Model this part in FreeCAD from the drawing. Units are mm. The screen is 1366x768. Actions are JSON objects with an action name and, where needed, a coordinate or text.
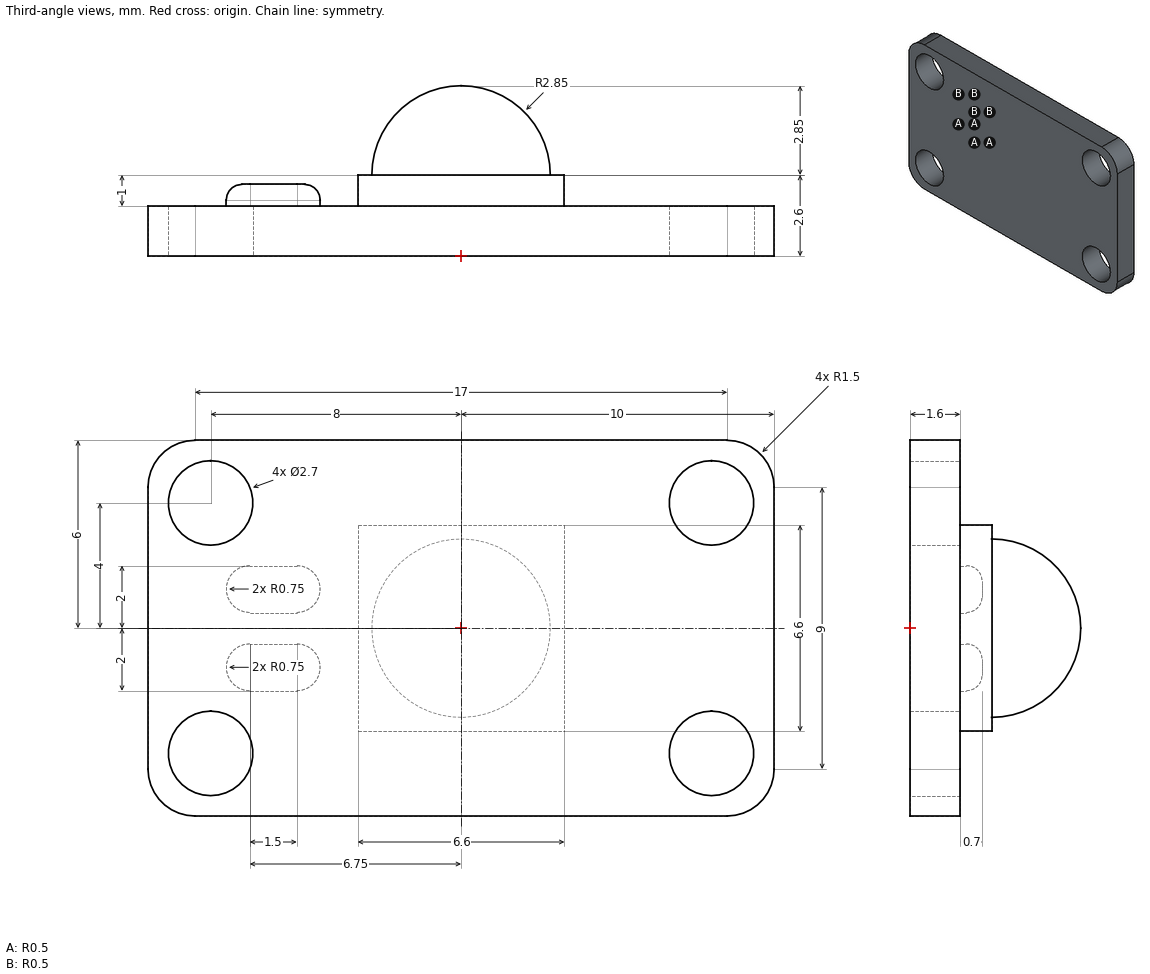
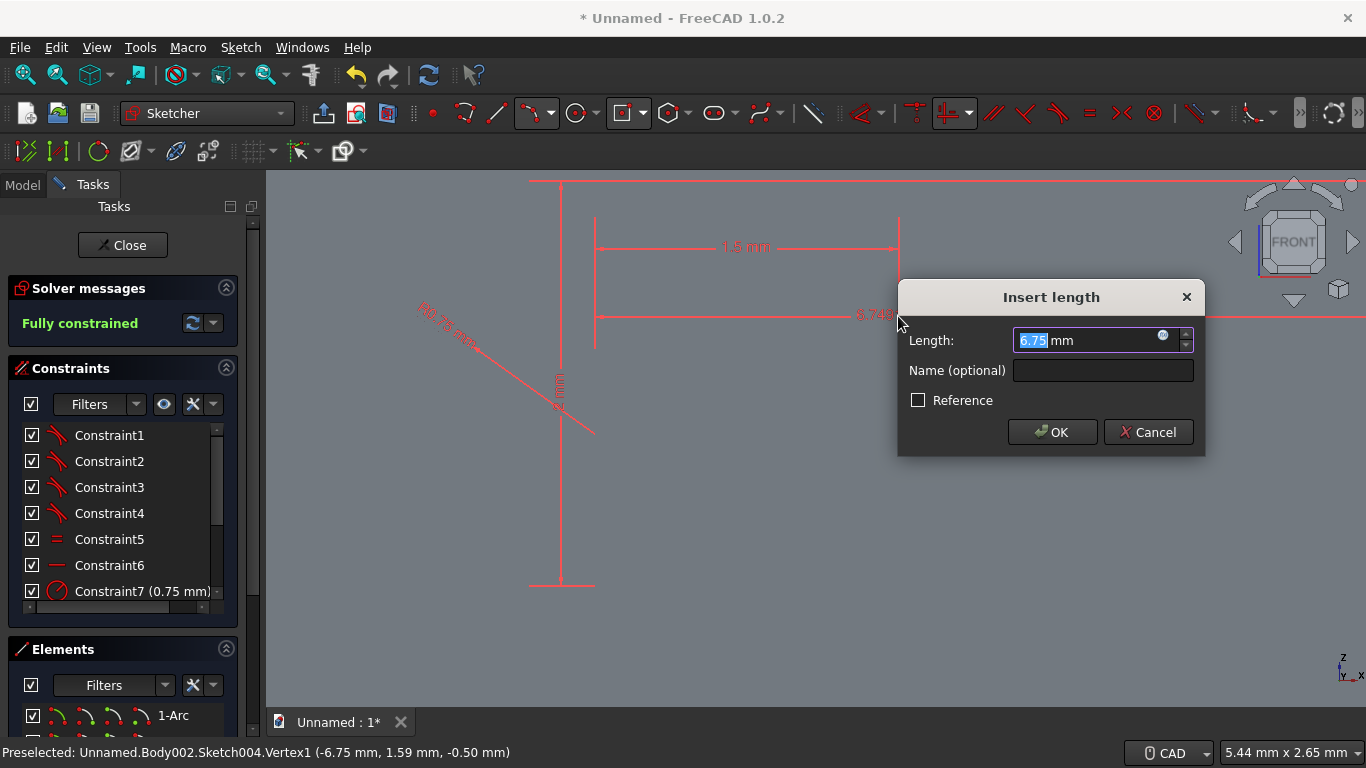
{"action": "type", "text": "6.75"}
{"action": "key", "text": "Return"}
{"action": "key", "text": "Escape"}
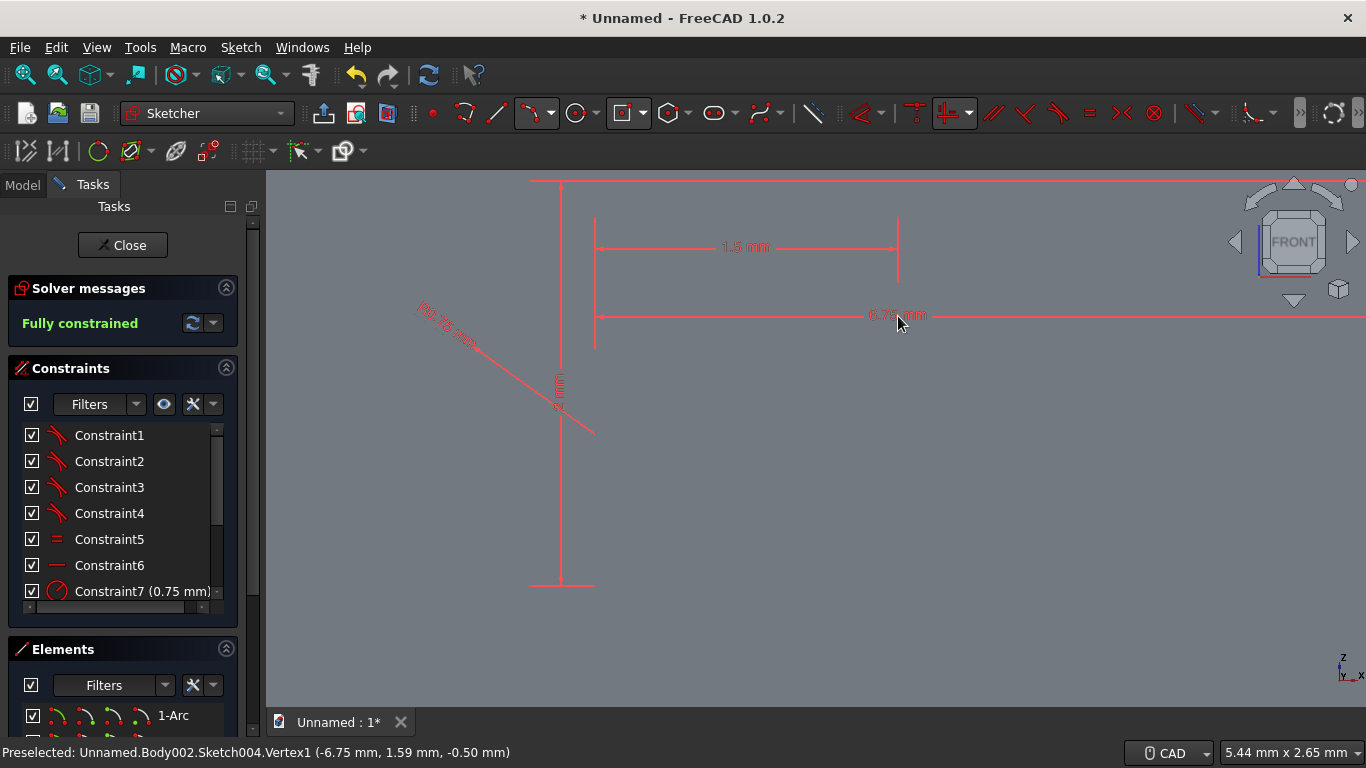
{"action": "left_click", "coordinate": [123, 245]}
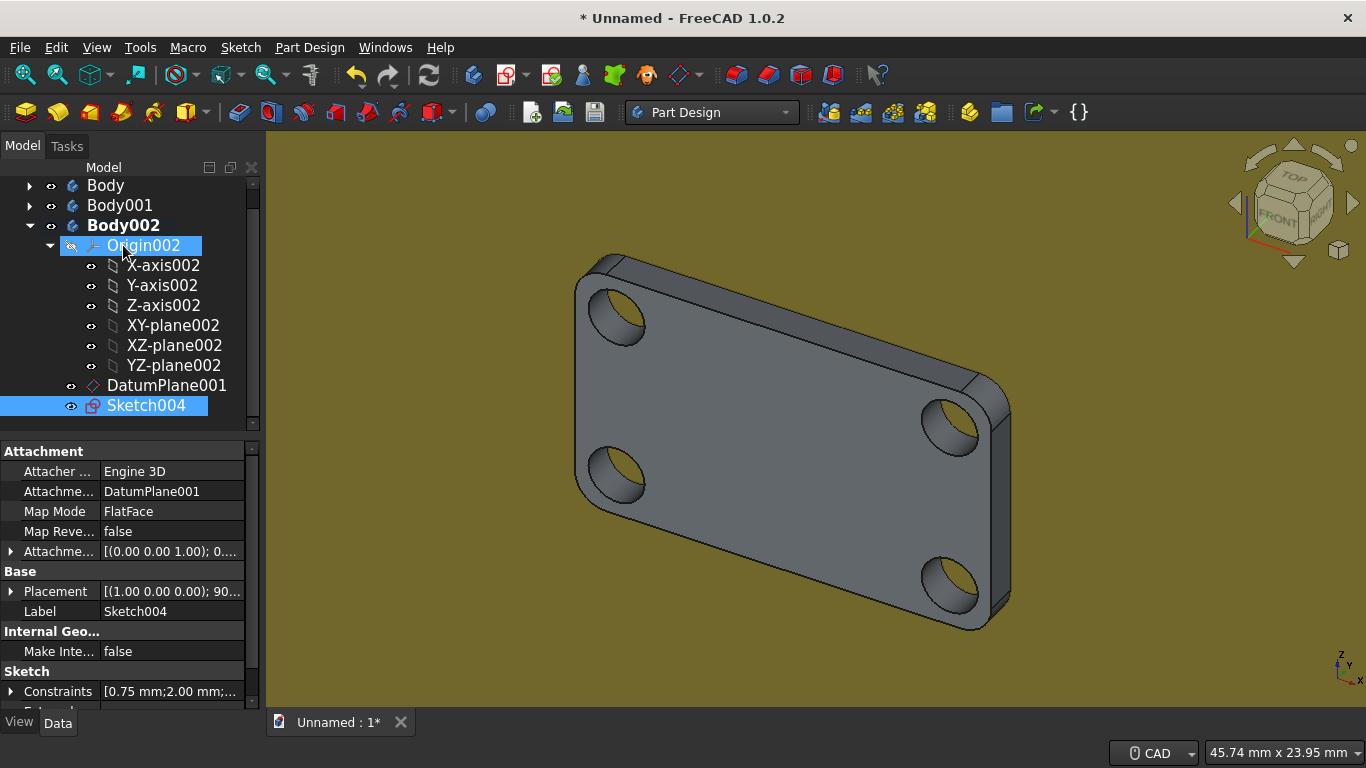
{"action": "left_click", "coordinate": [26, 112]}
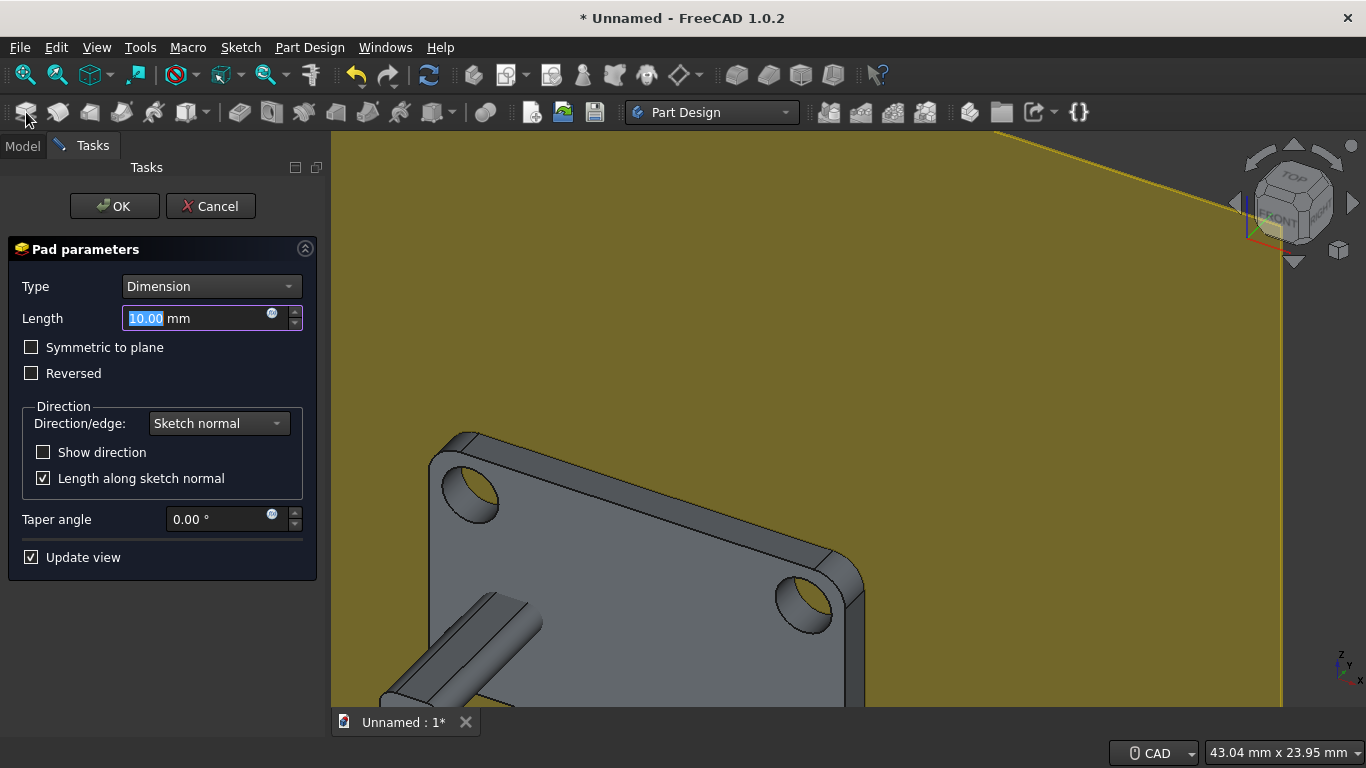
{"action": "type", "text": "0.7"}
{"action": "key", "text": "Tab"}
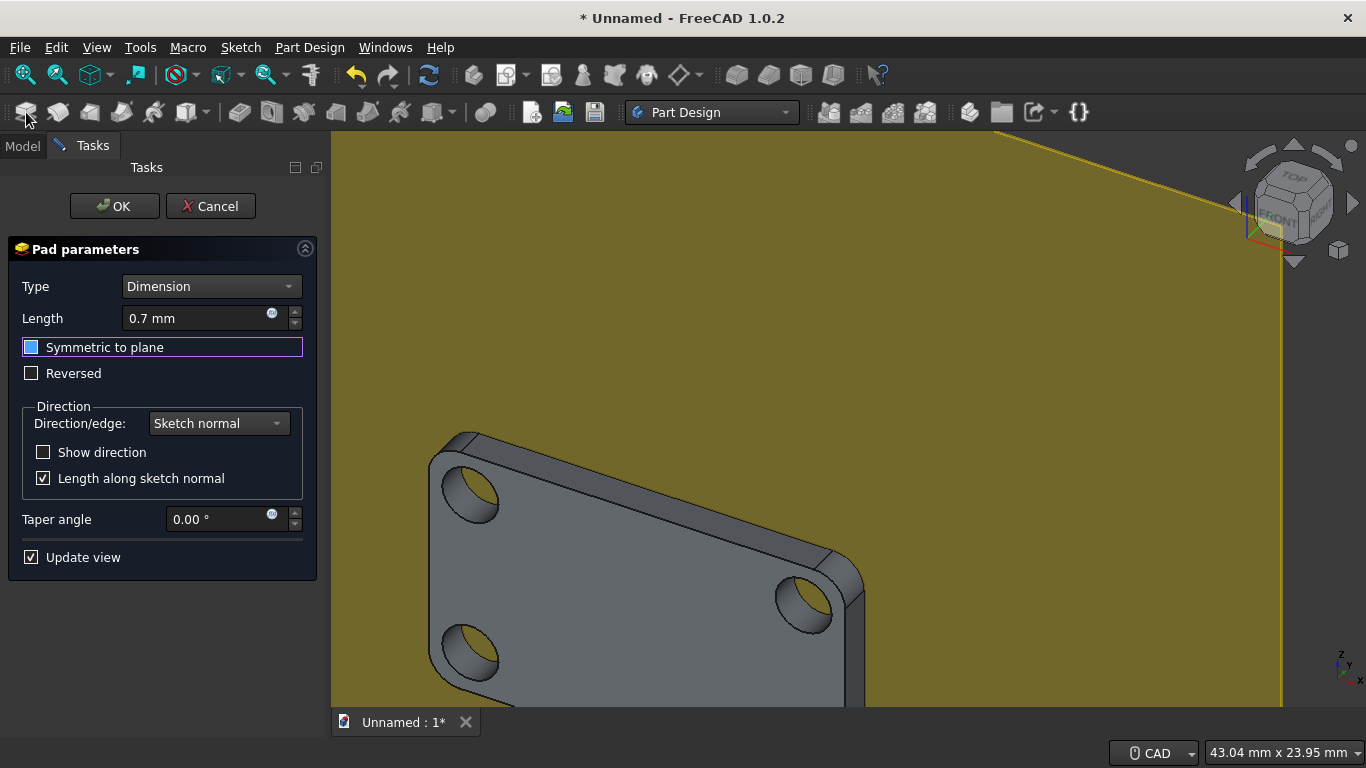
{"action": "left_click", "coordinate": [30, 373]}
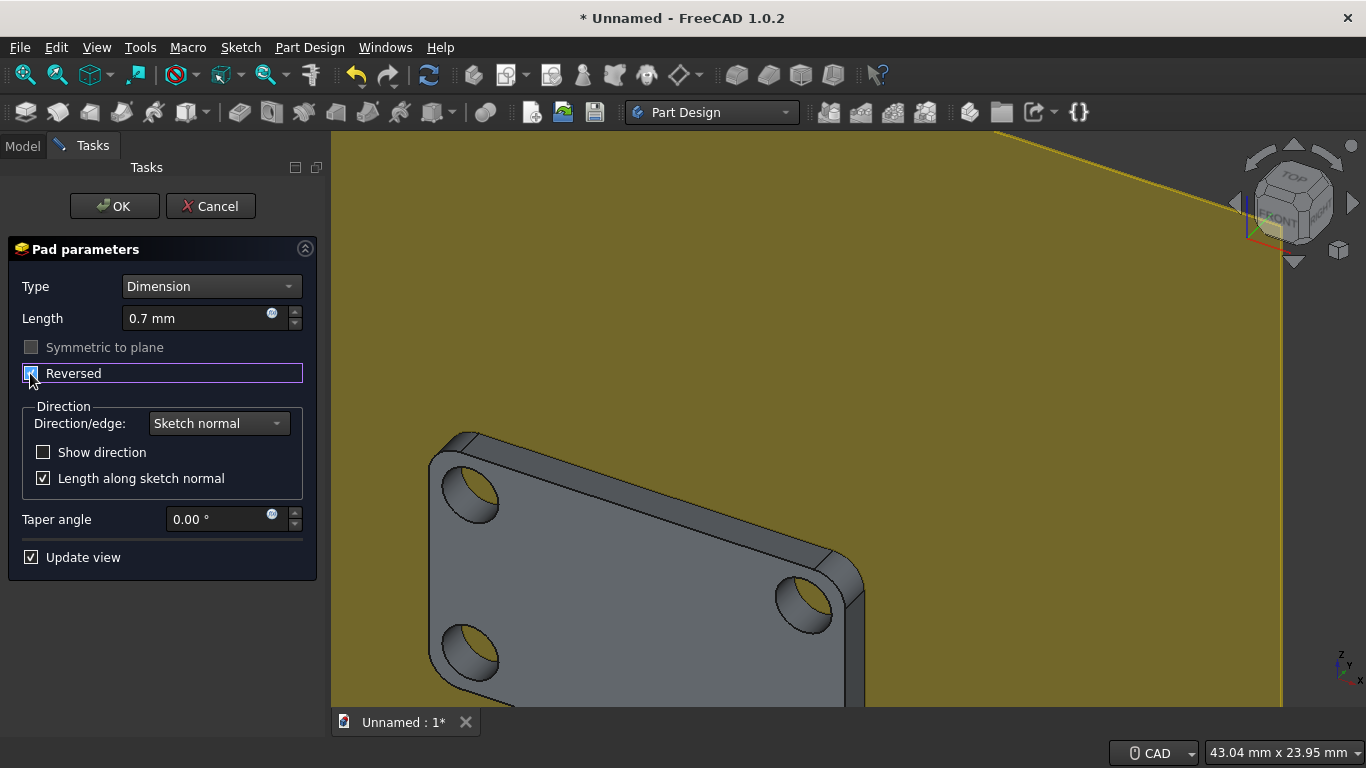
{"action": "left_click", "coordinate": [115, 206]}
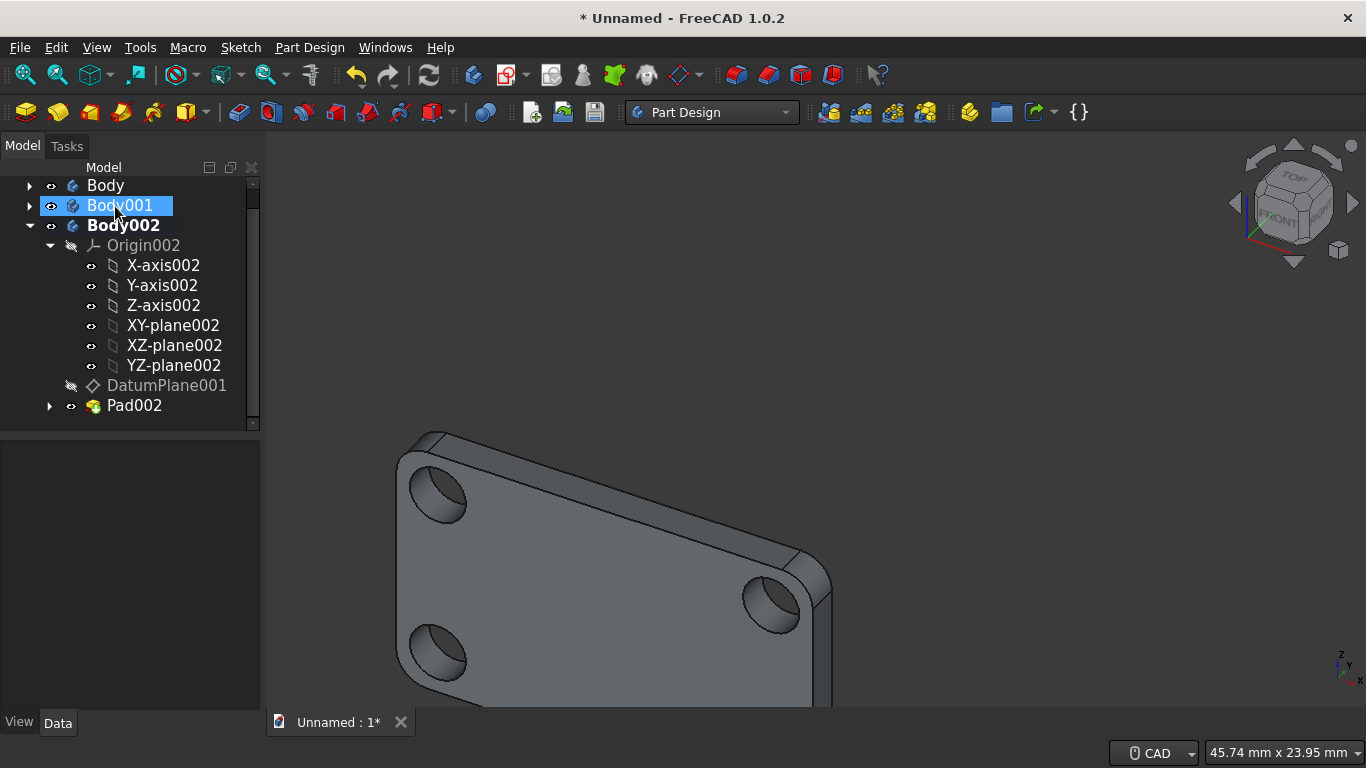
{"action": "key", "text": "v f"}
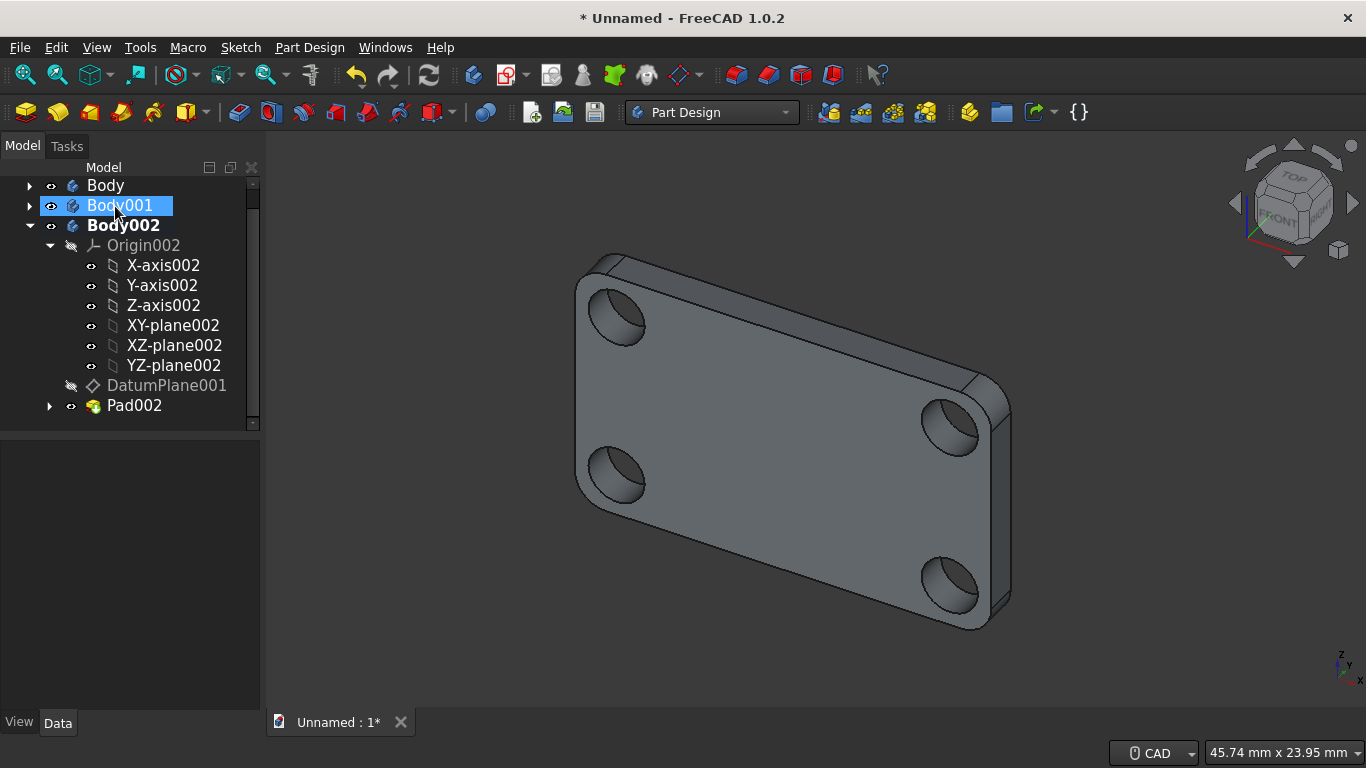
{"action": "key", "text": "0"}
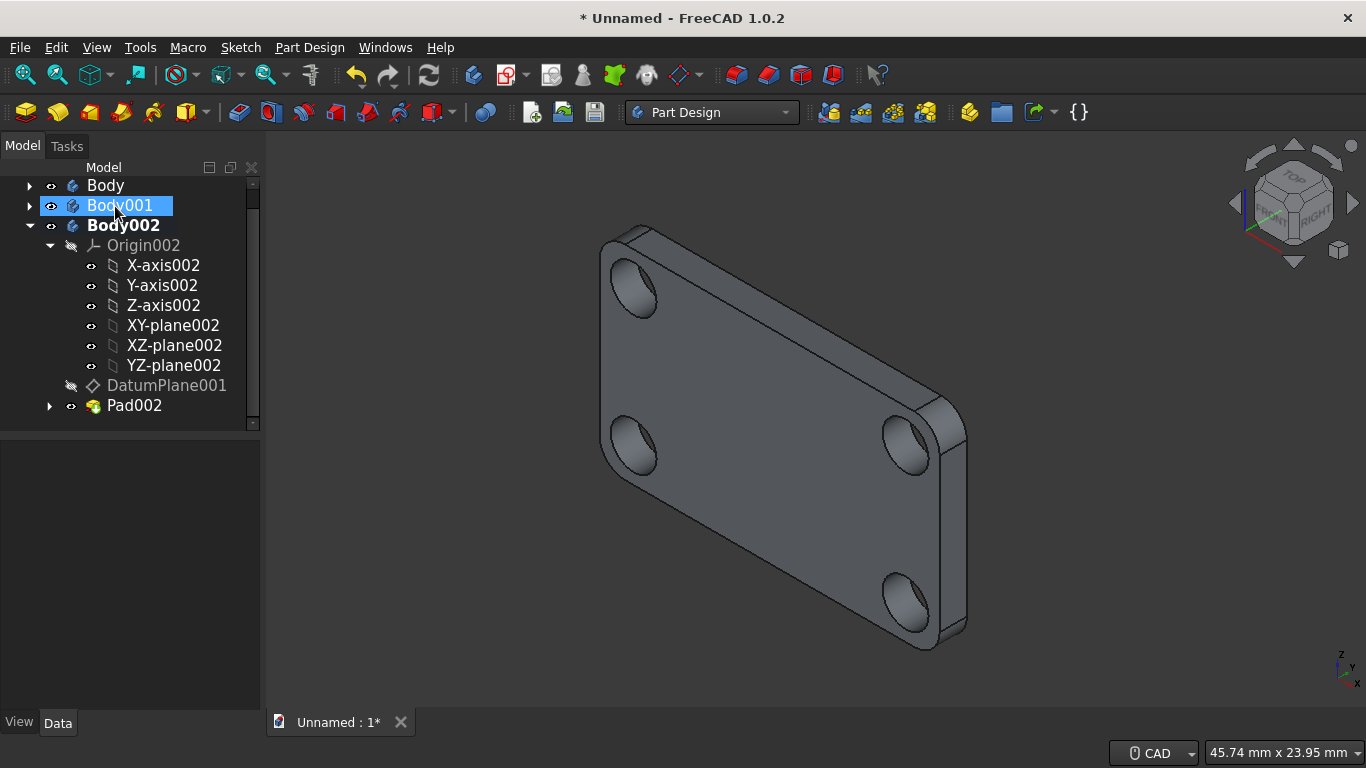
{"action": "key", "text": "v f"}